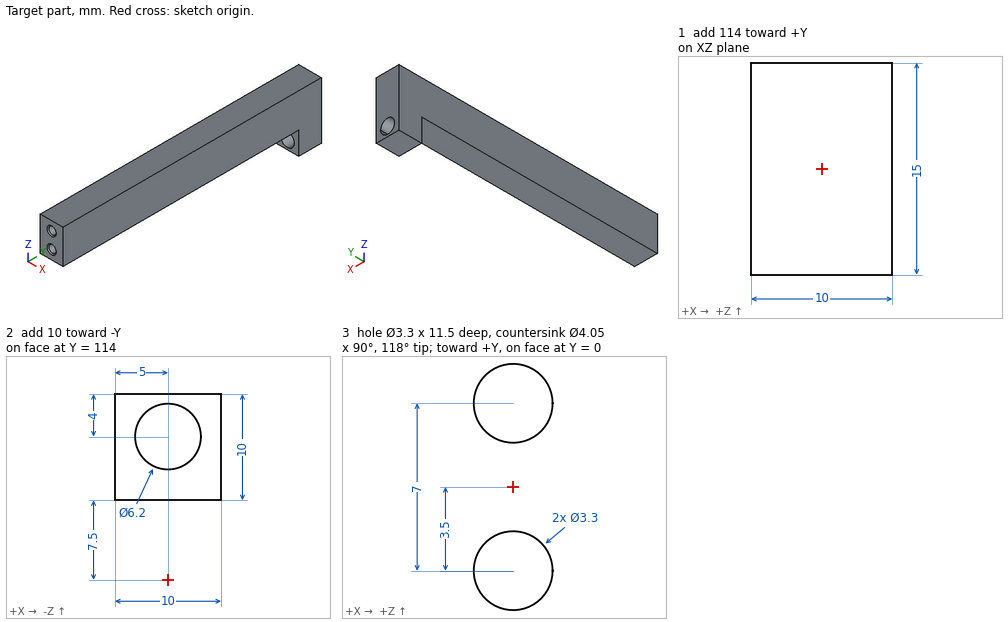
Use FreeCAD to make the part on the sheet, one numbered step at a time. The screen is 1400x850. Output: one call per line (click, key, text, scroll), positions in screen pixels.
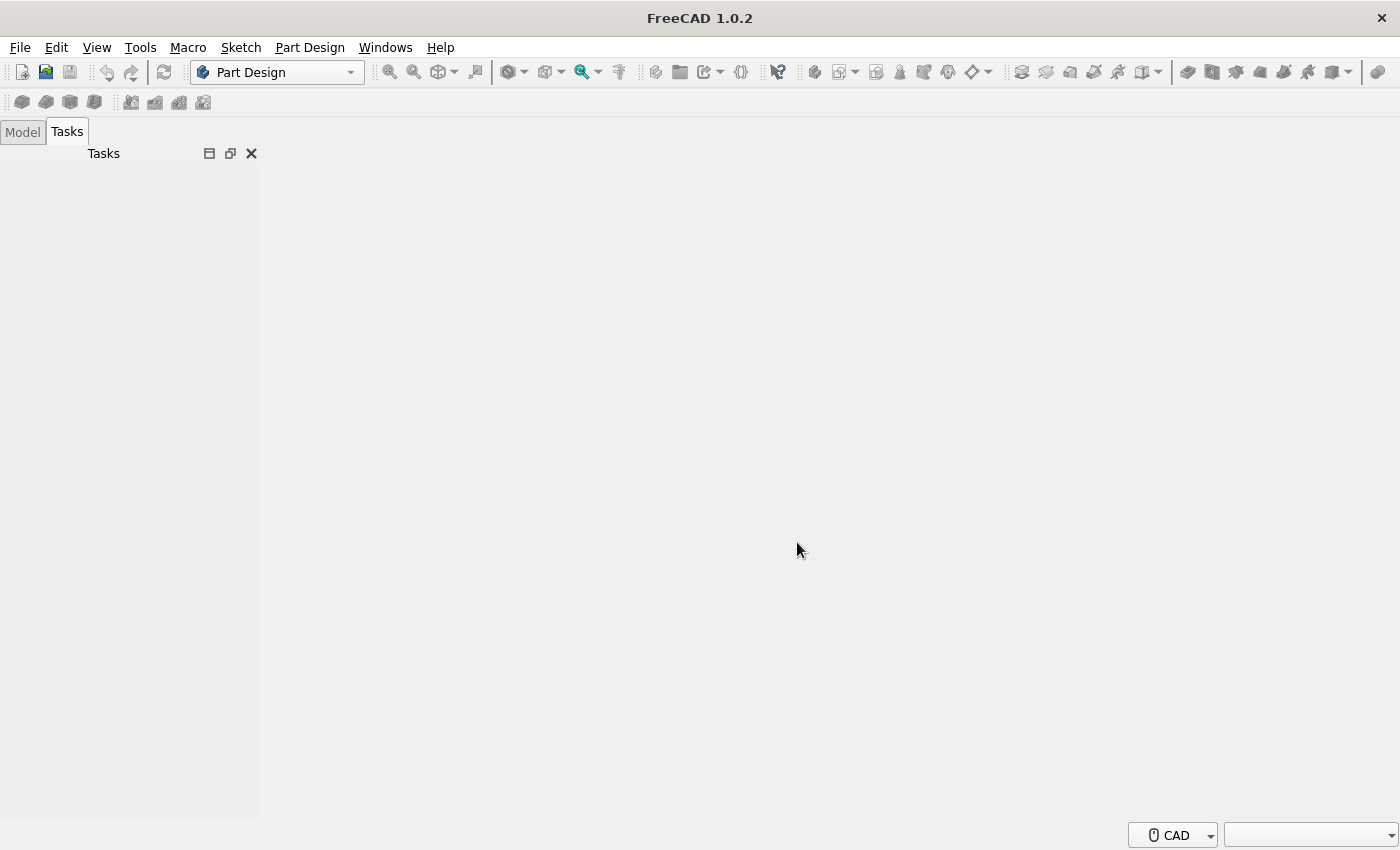
click(22, 72)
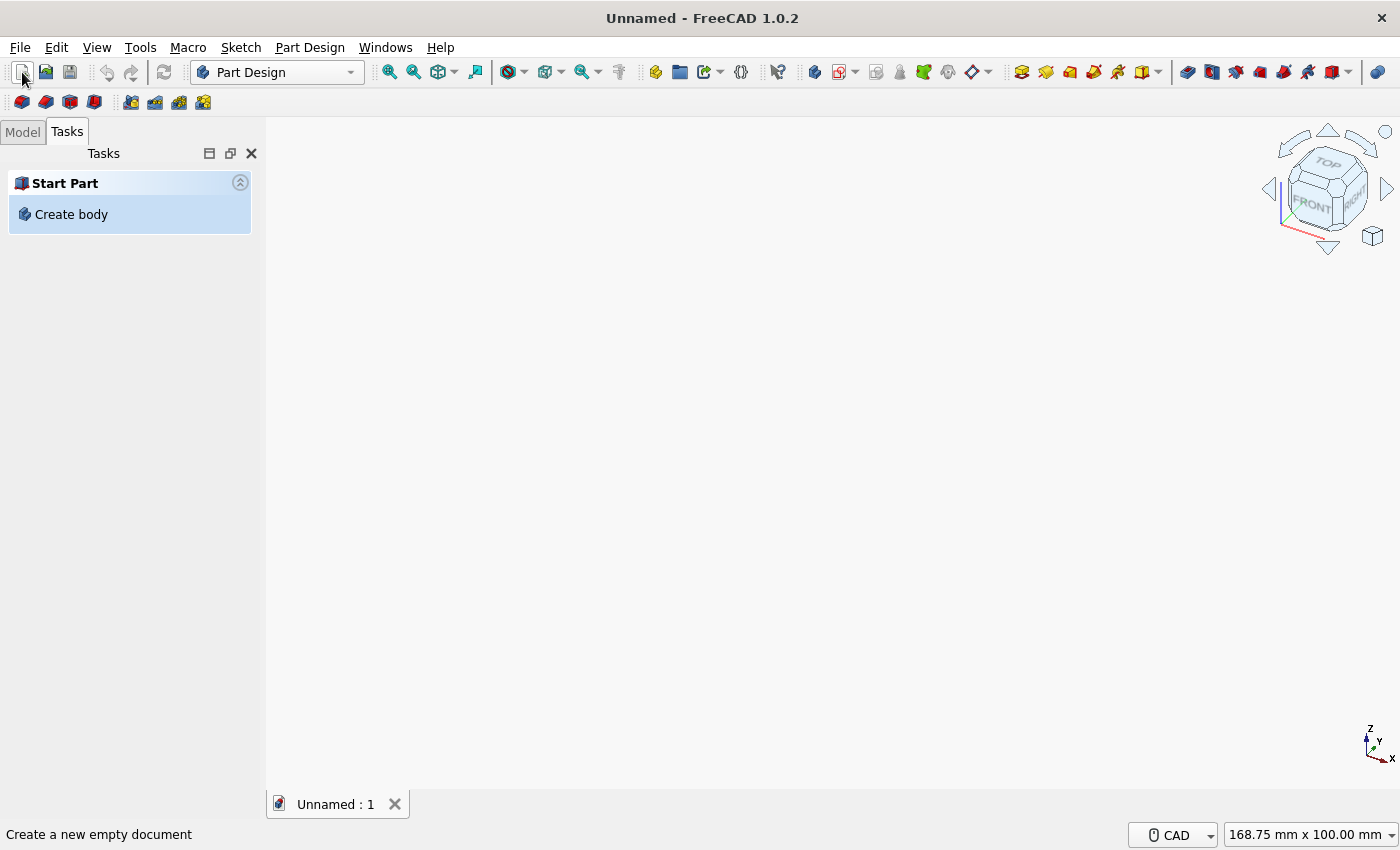
click(840, 72)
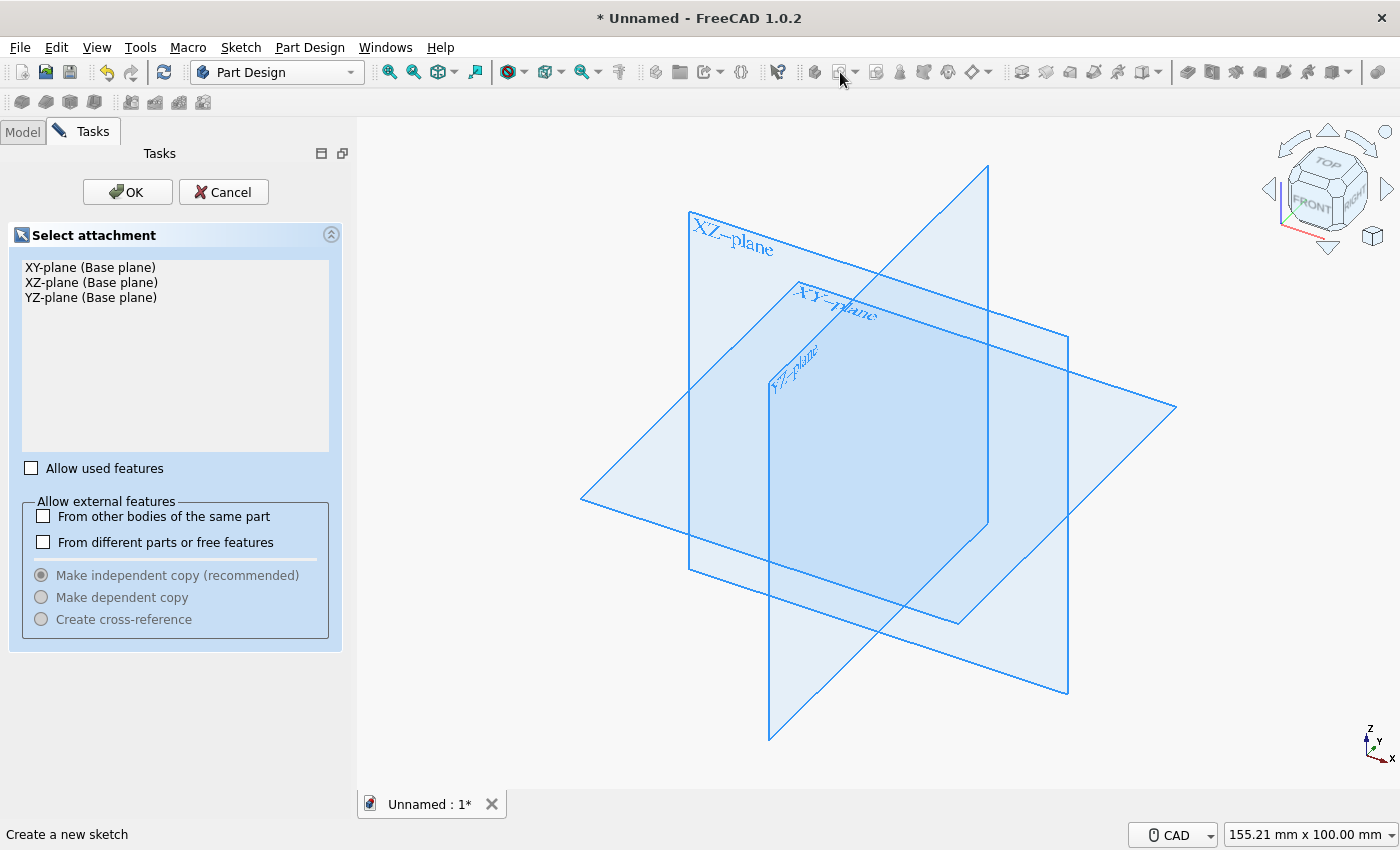
click(82, 282)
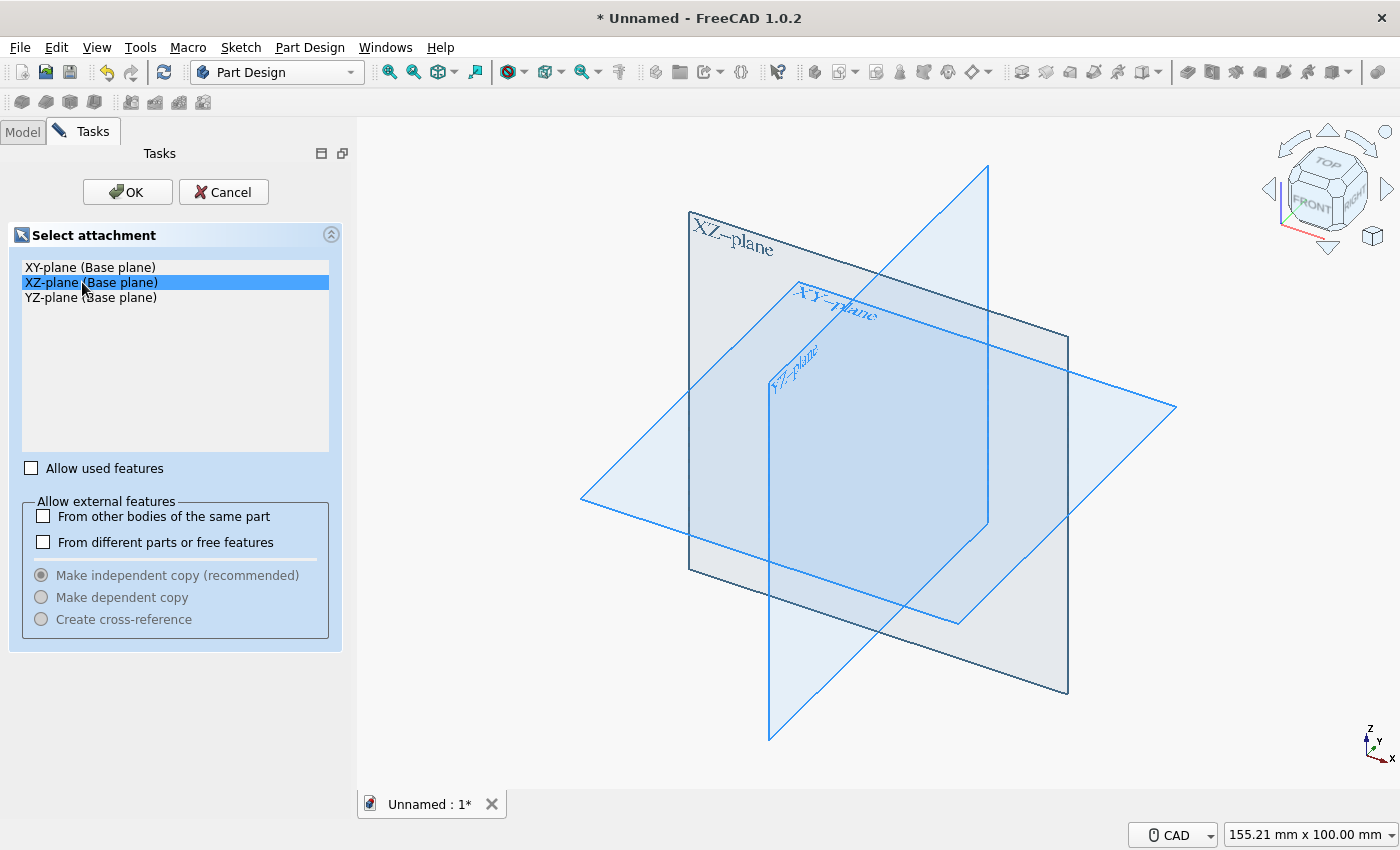
click(128, 192)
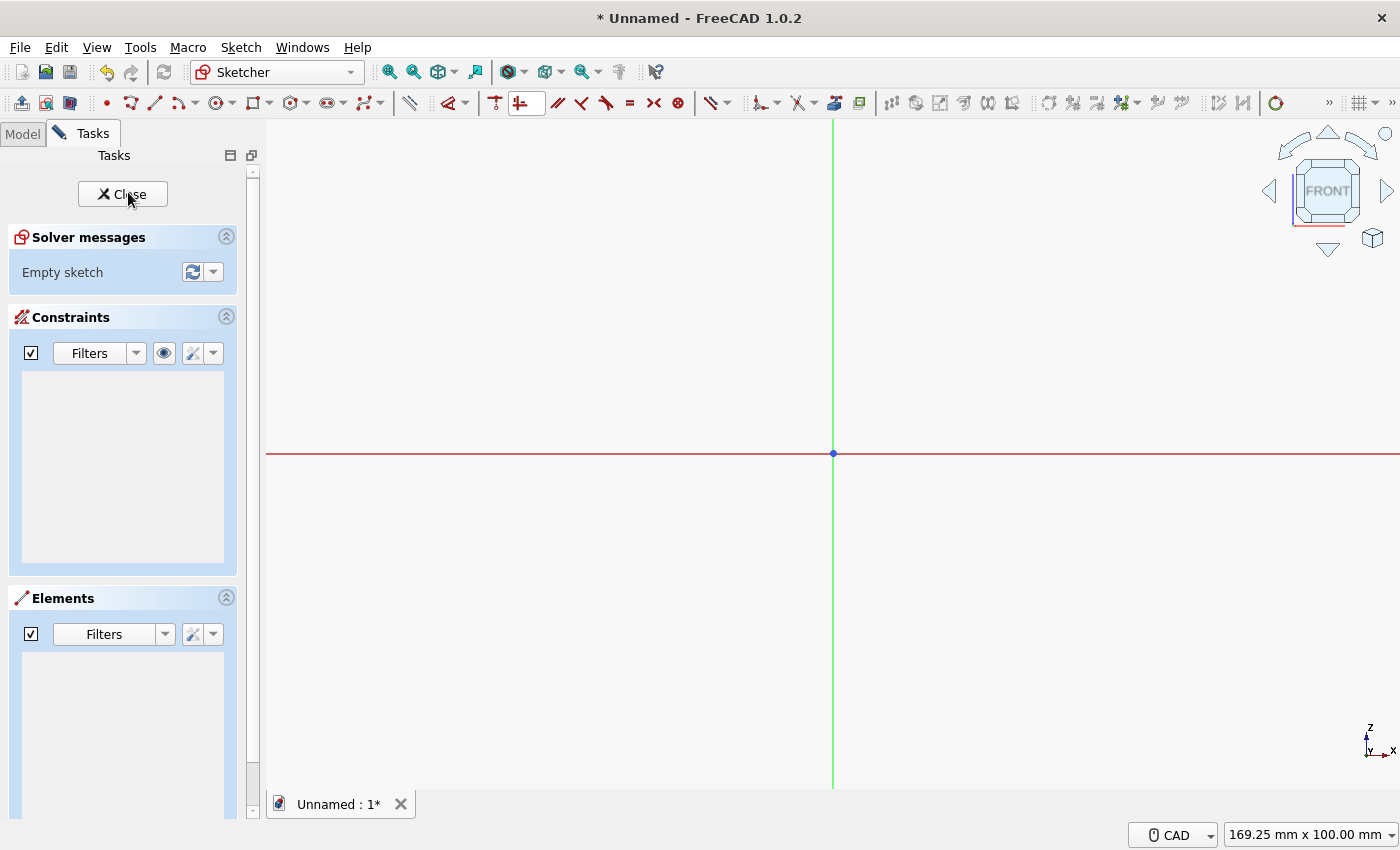
scroll(855, 454, up, 7)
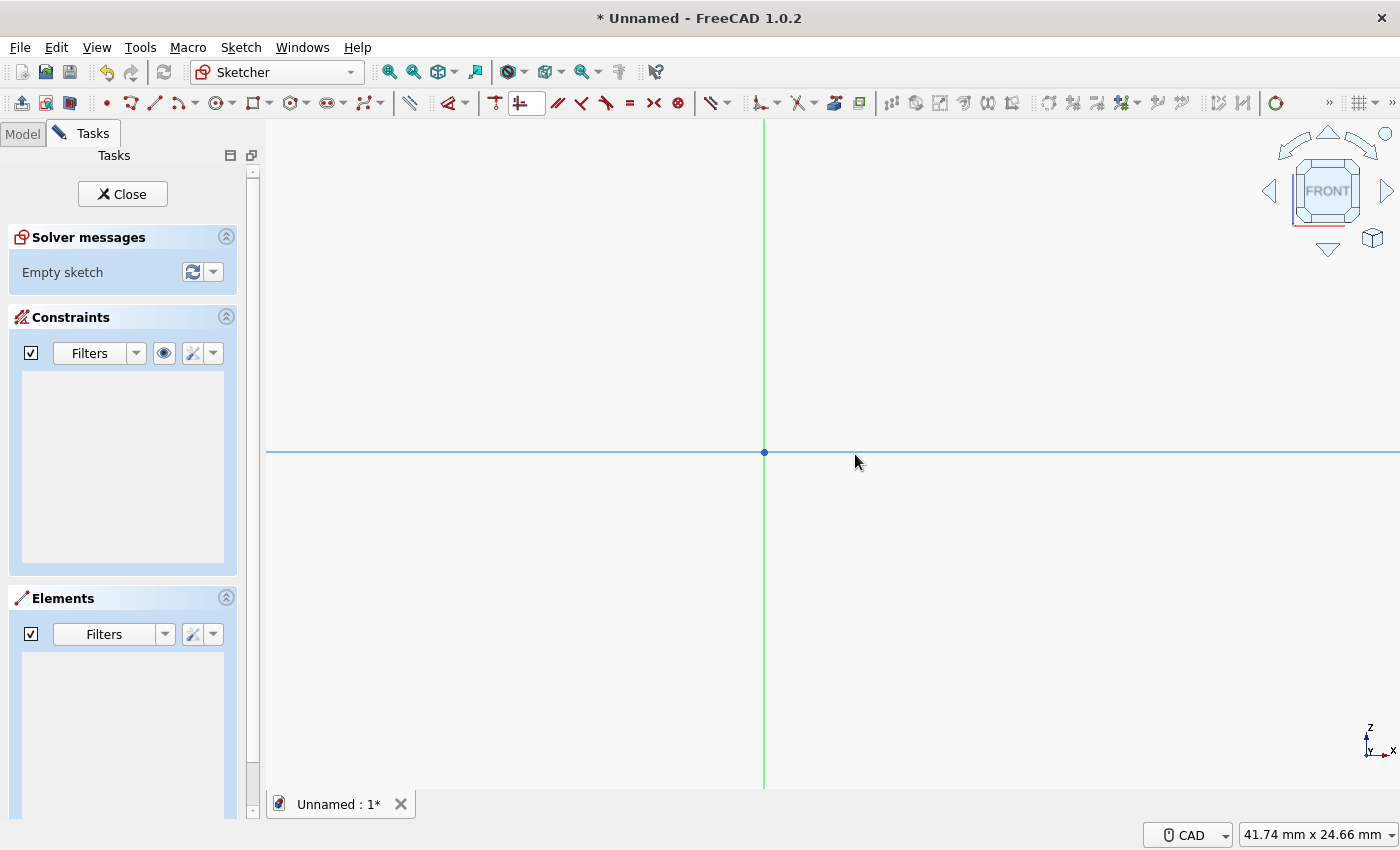
click(272, 104)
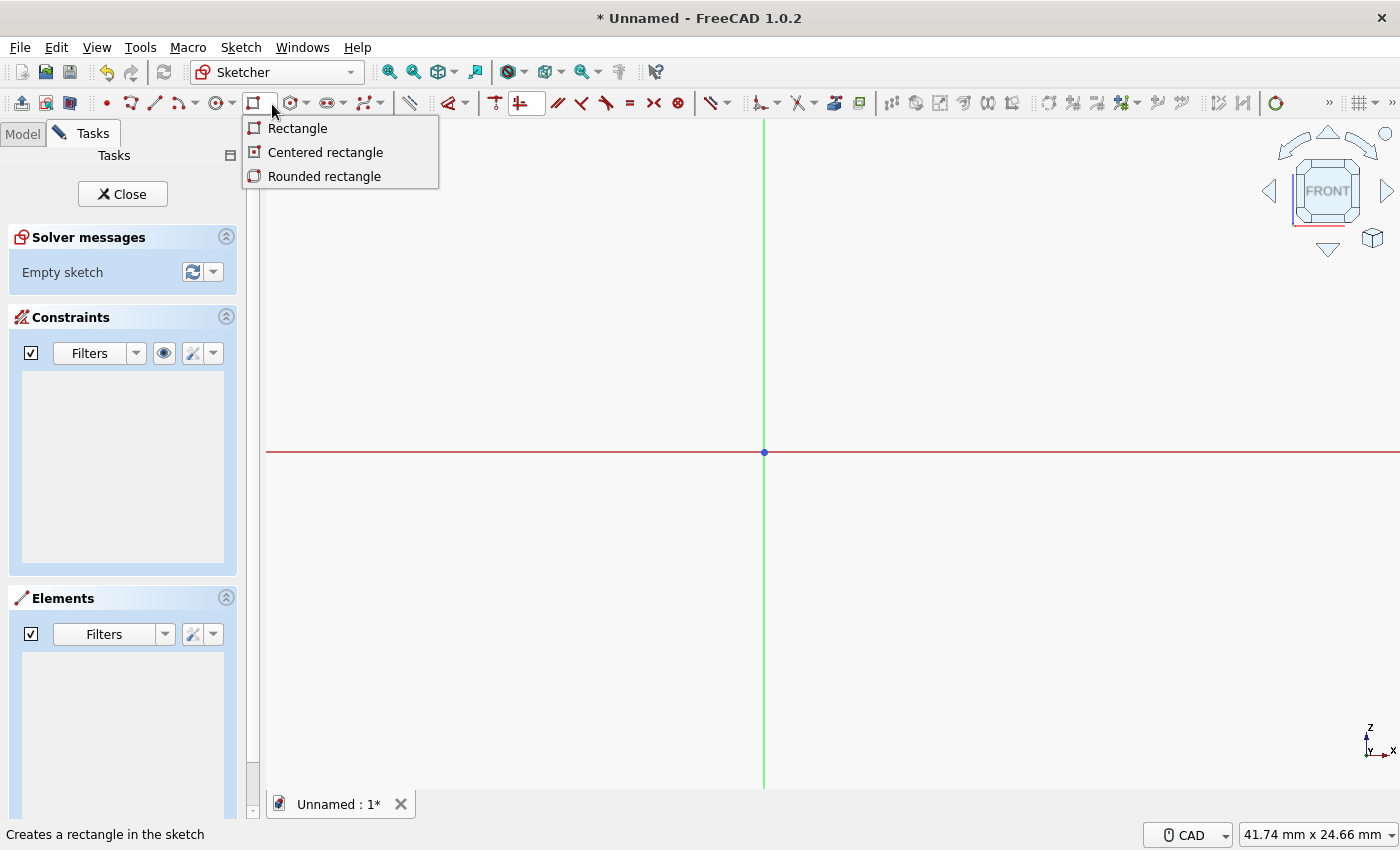
click(340, 152)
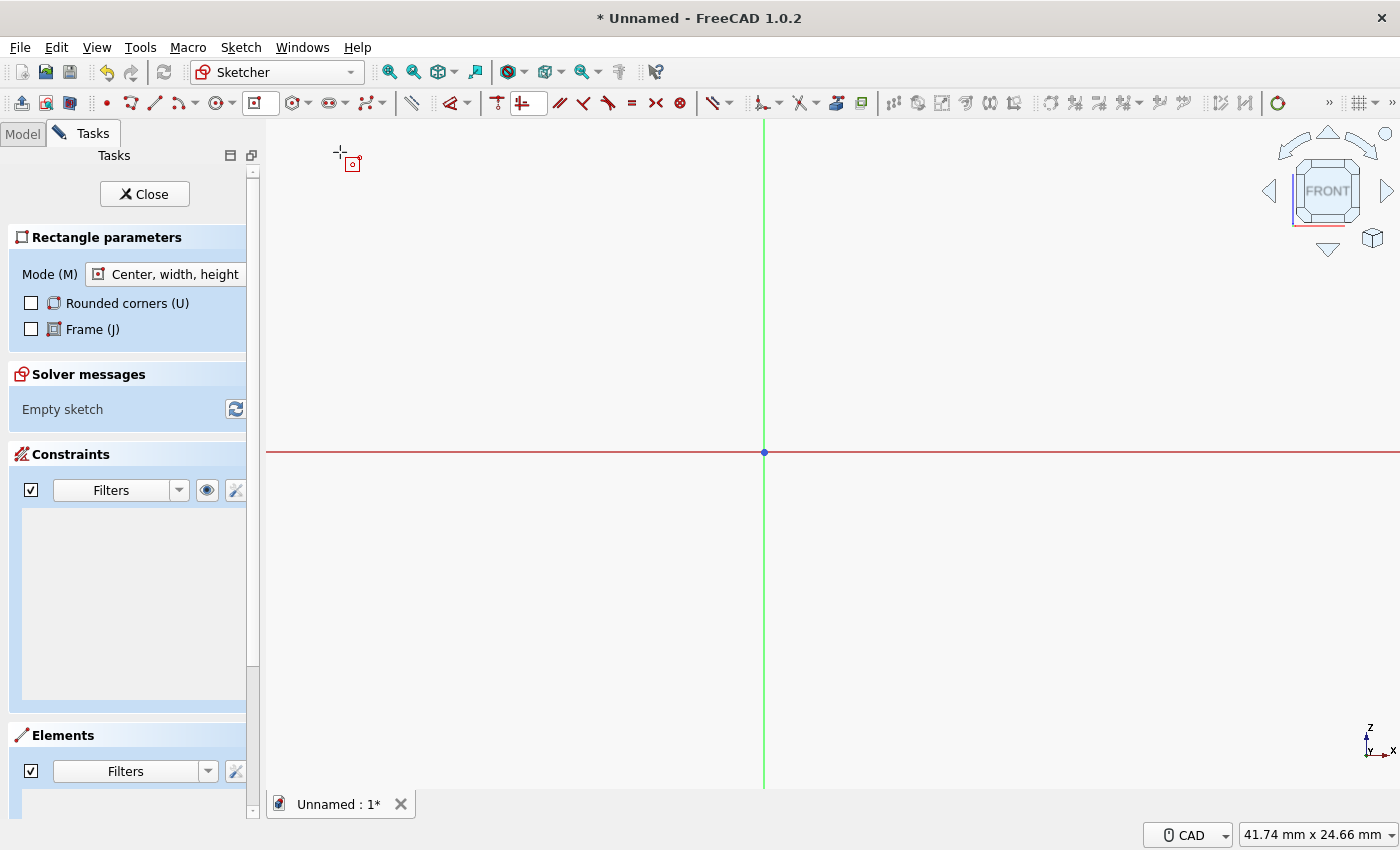
click(764, 452)
move(900, 249)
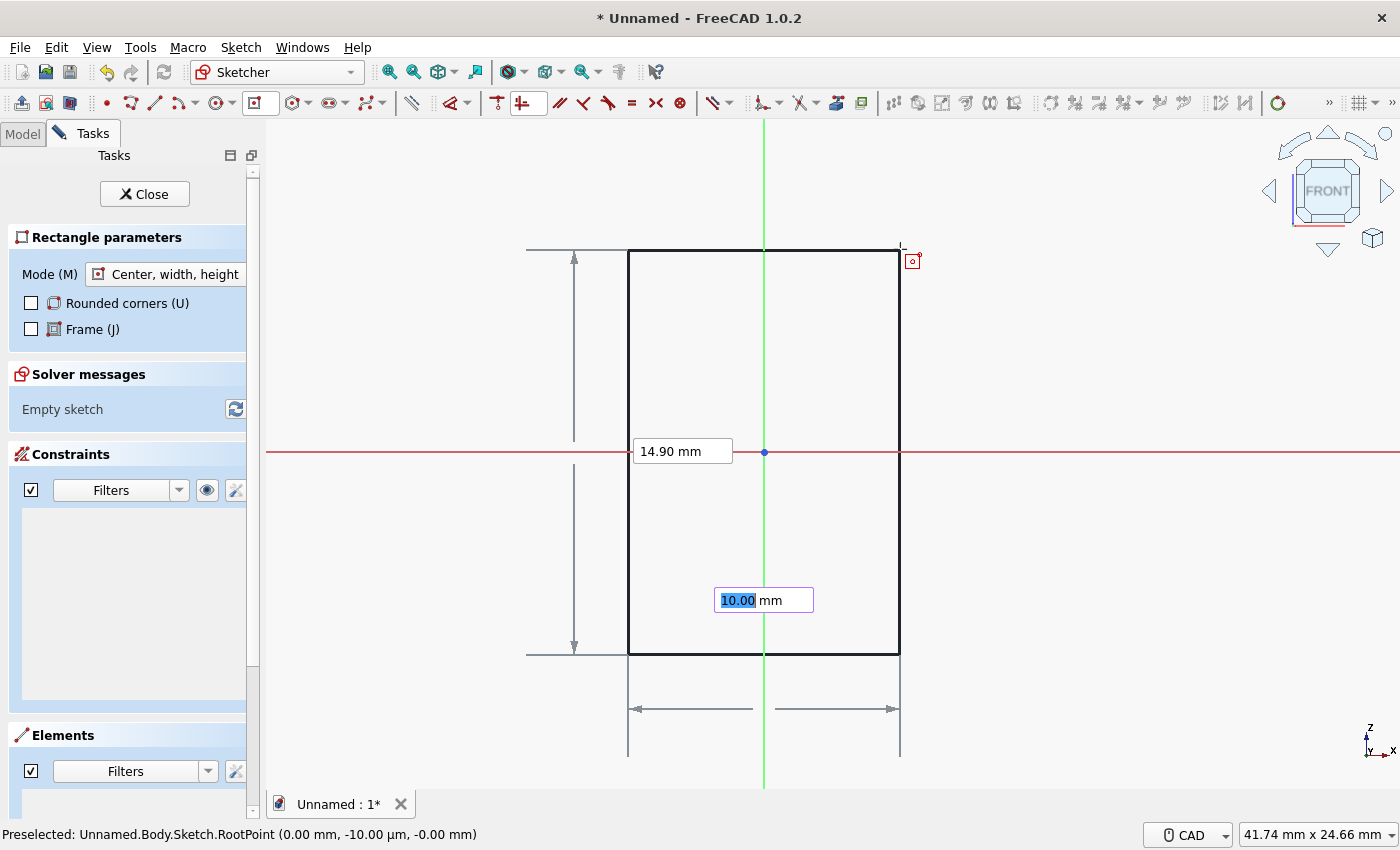
text(10)
key(Tab)
text(15)
key(Return)
key(Escape)